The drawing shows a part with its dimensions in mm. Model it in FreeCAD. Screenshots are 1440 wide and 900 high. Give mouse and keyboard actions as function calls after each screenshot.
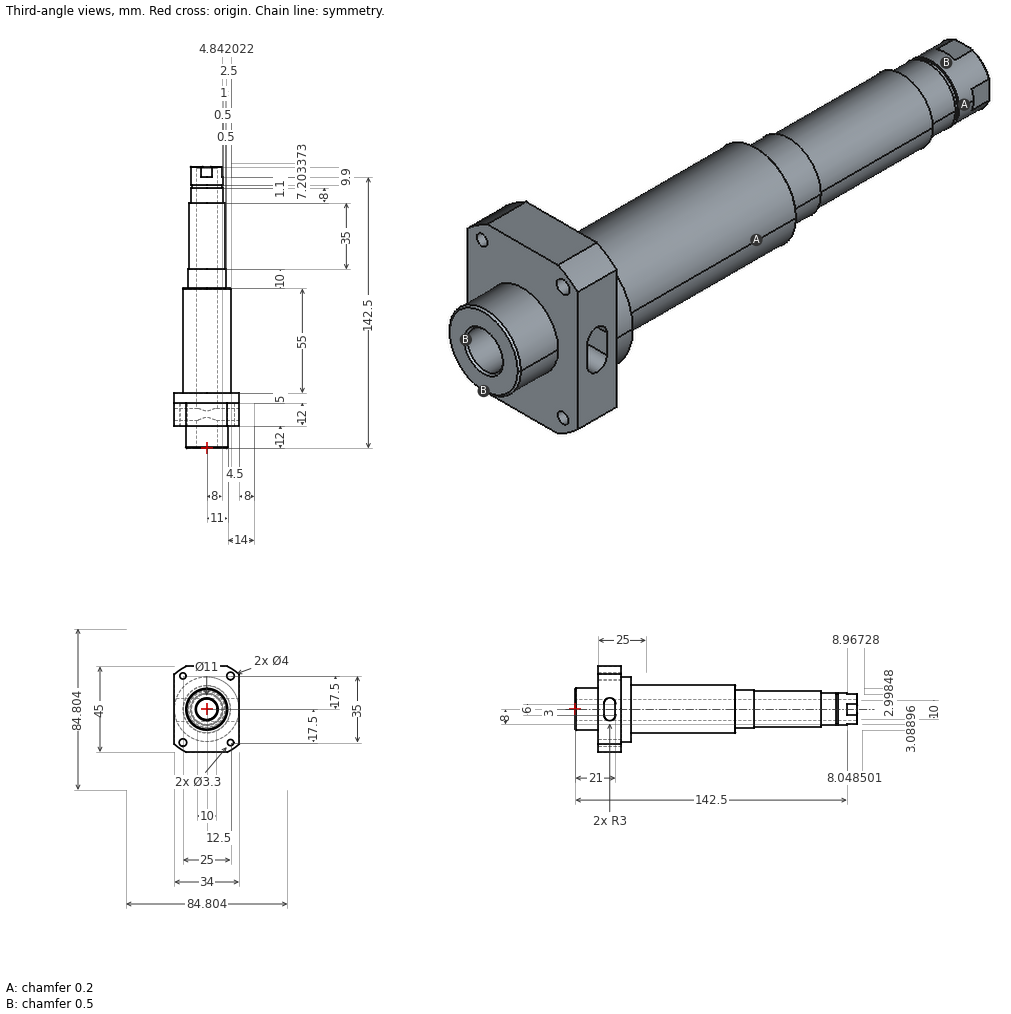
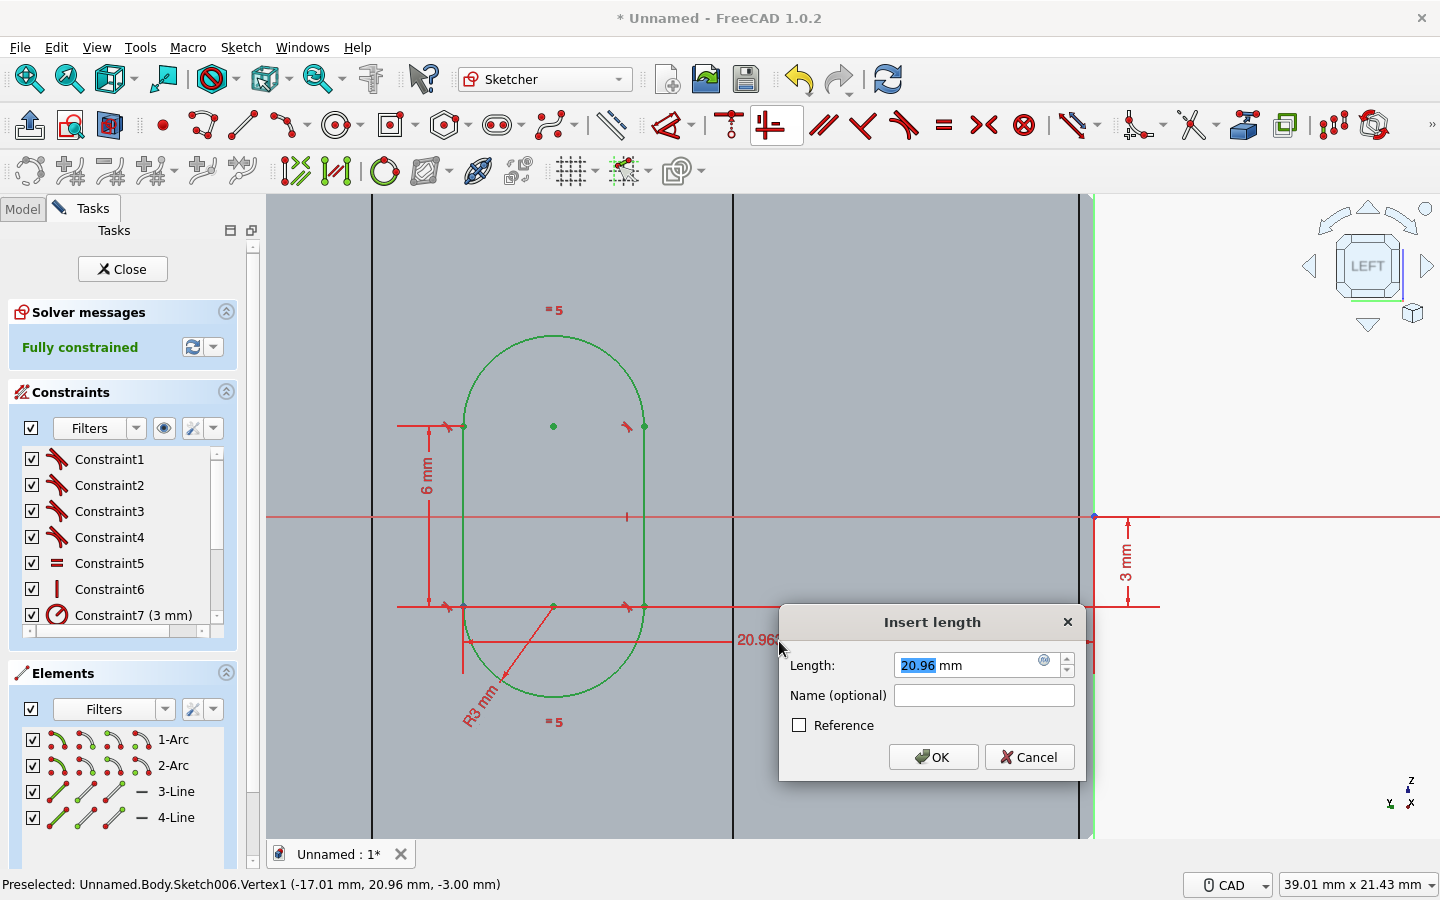
text(21)
key(Return)
key(Escape)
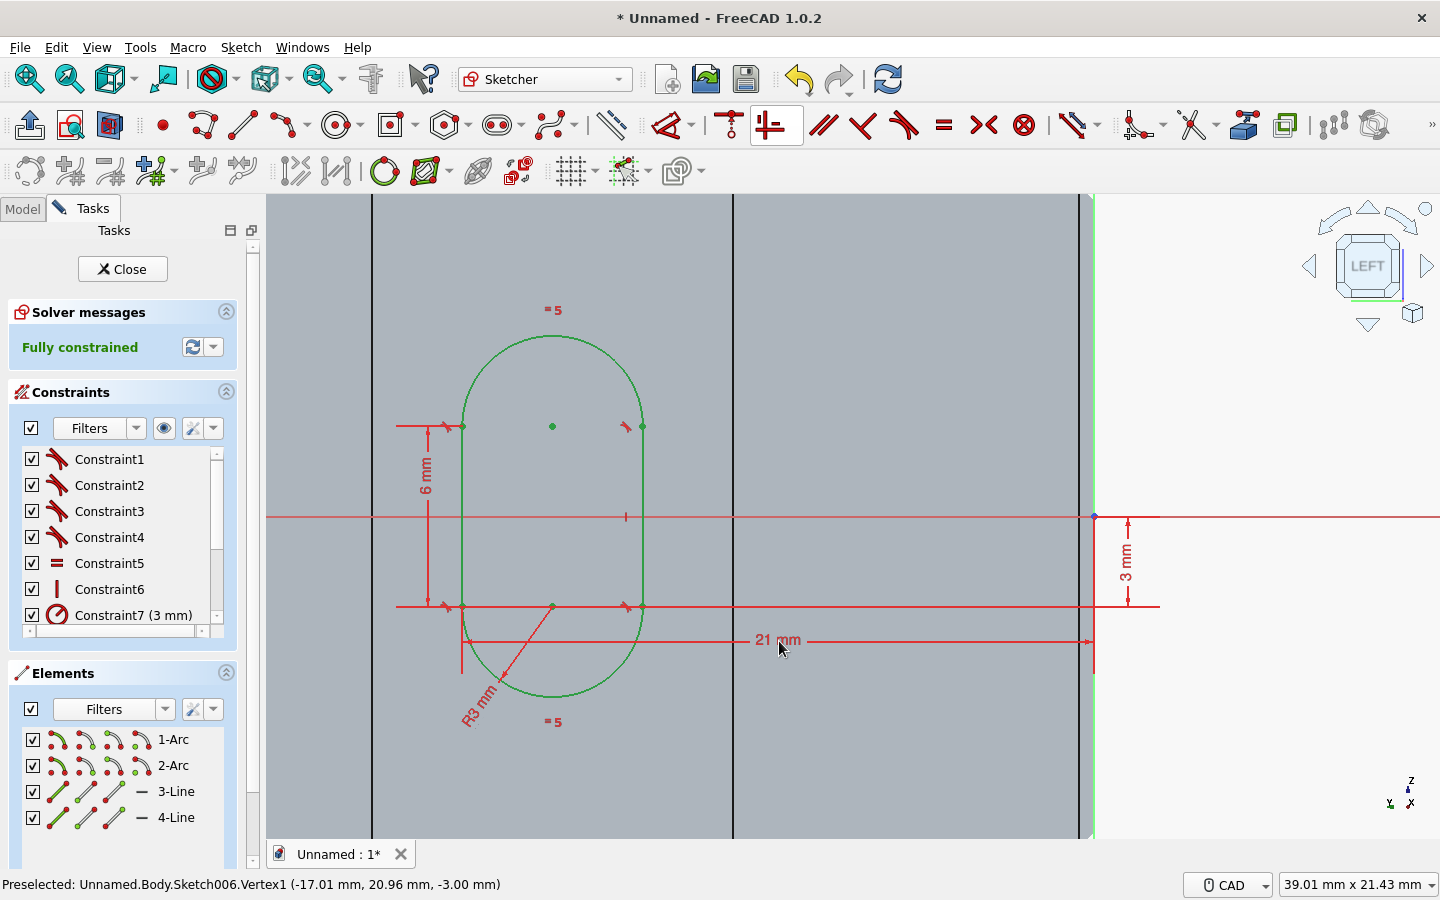
click(123, 269)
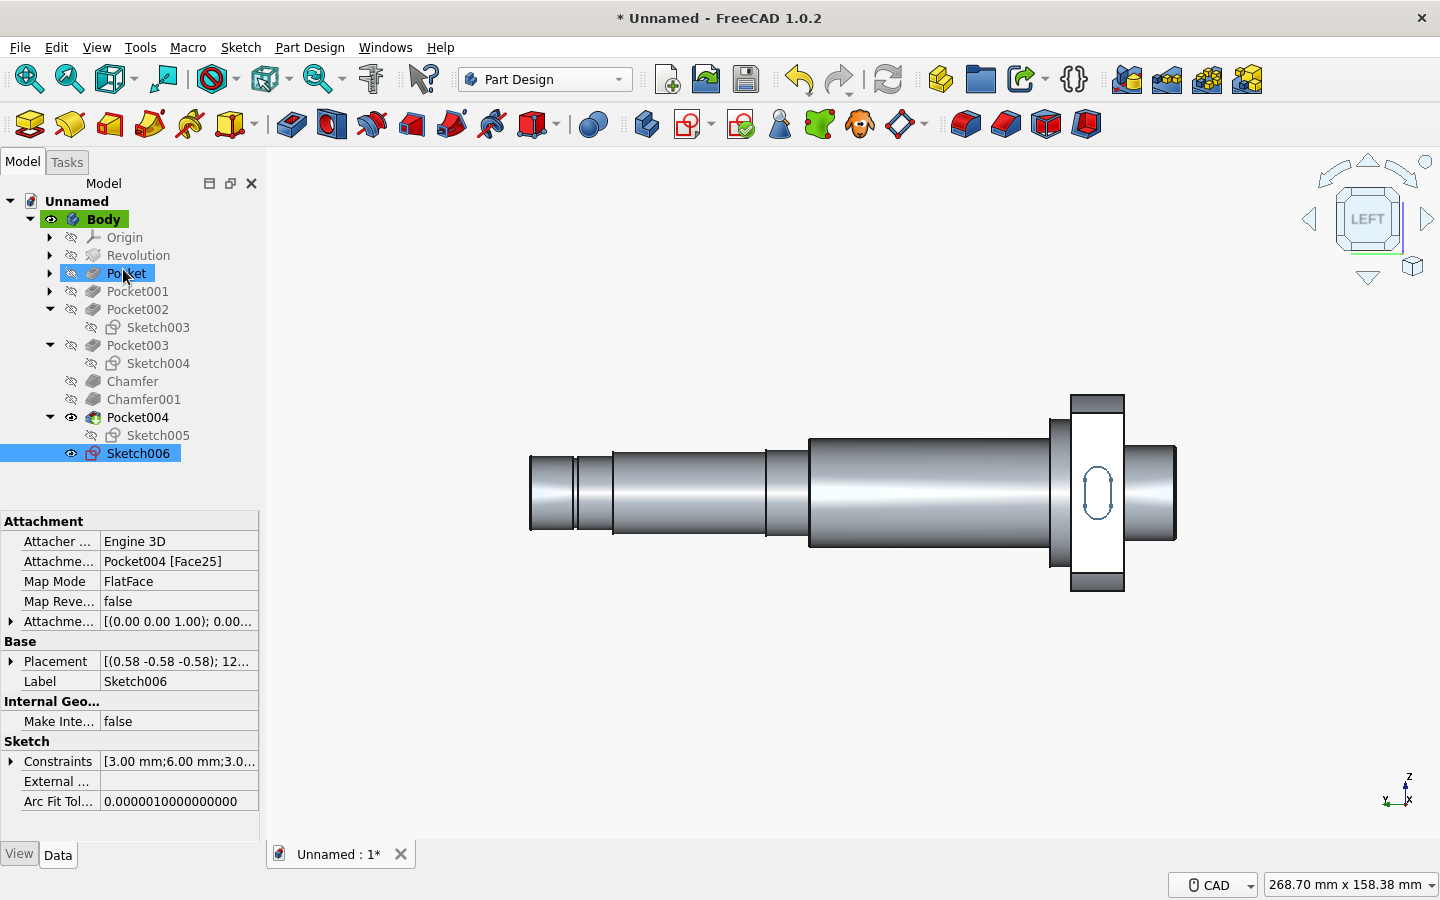
click(292, 124)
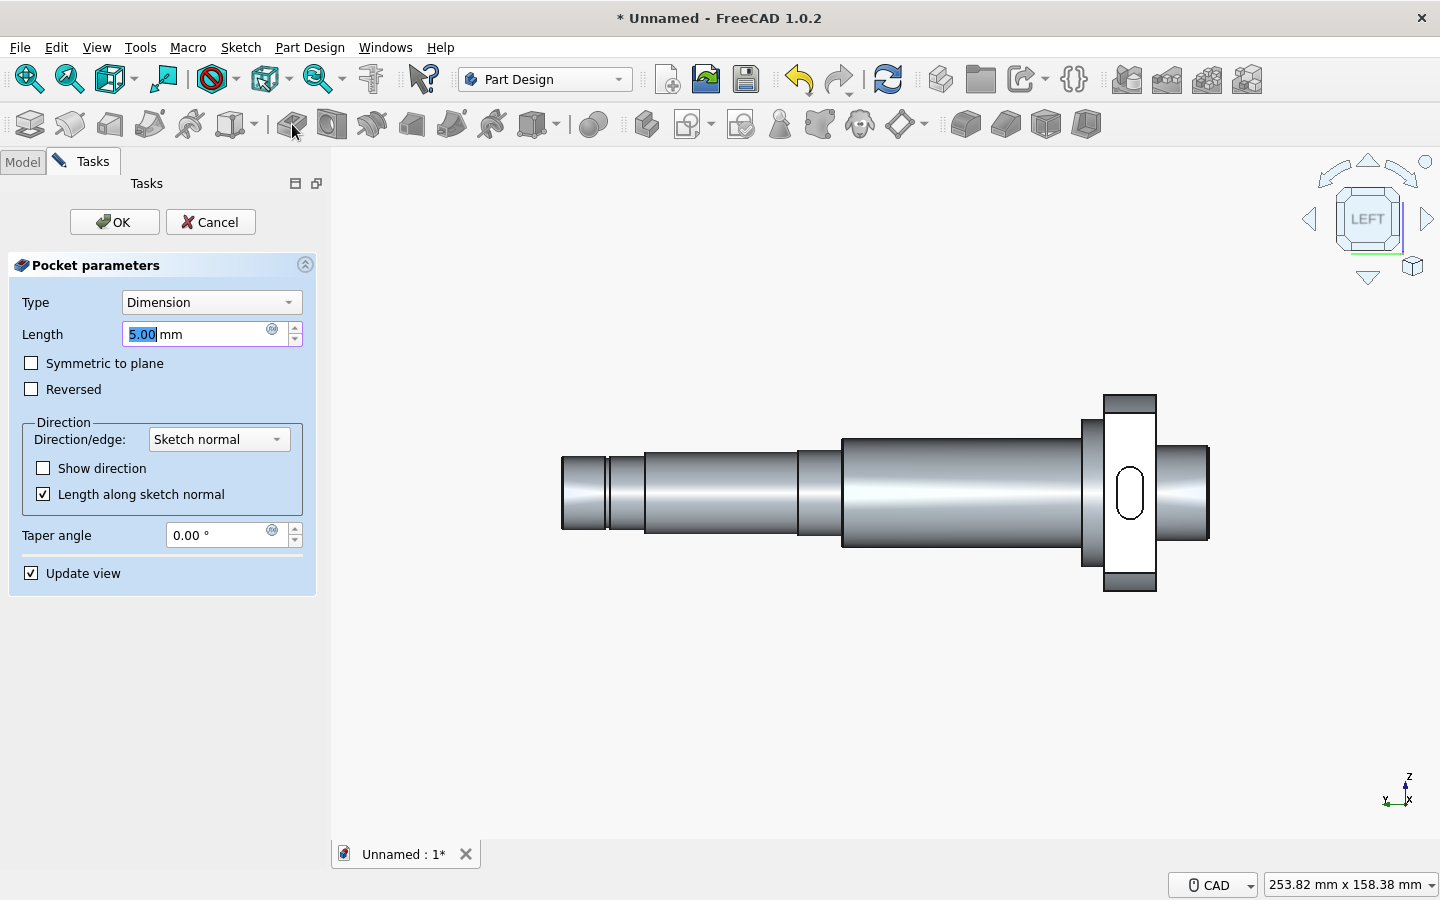
click(212, 302)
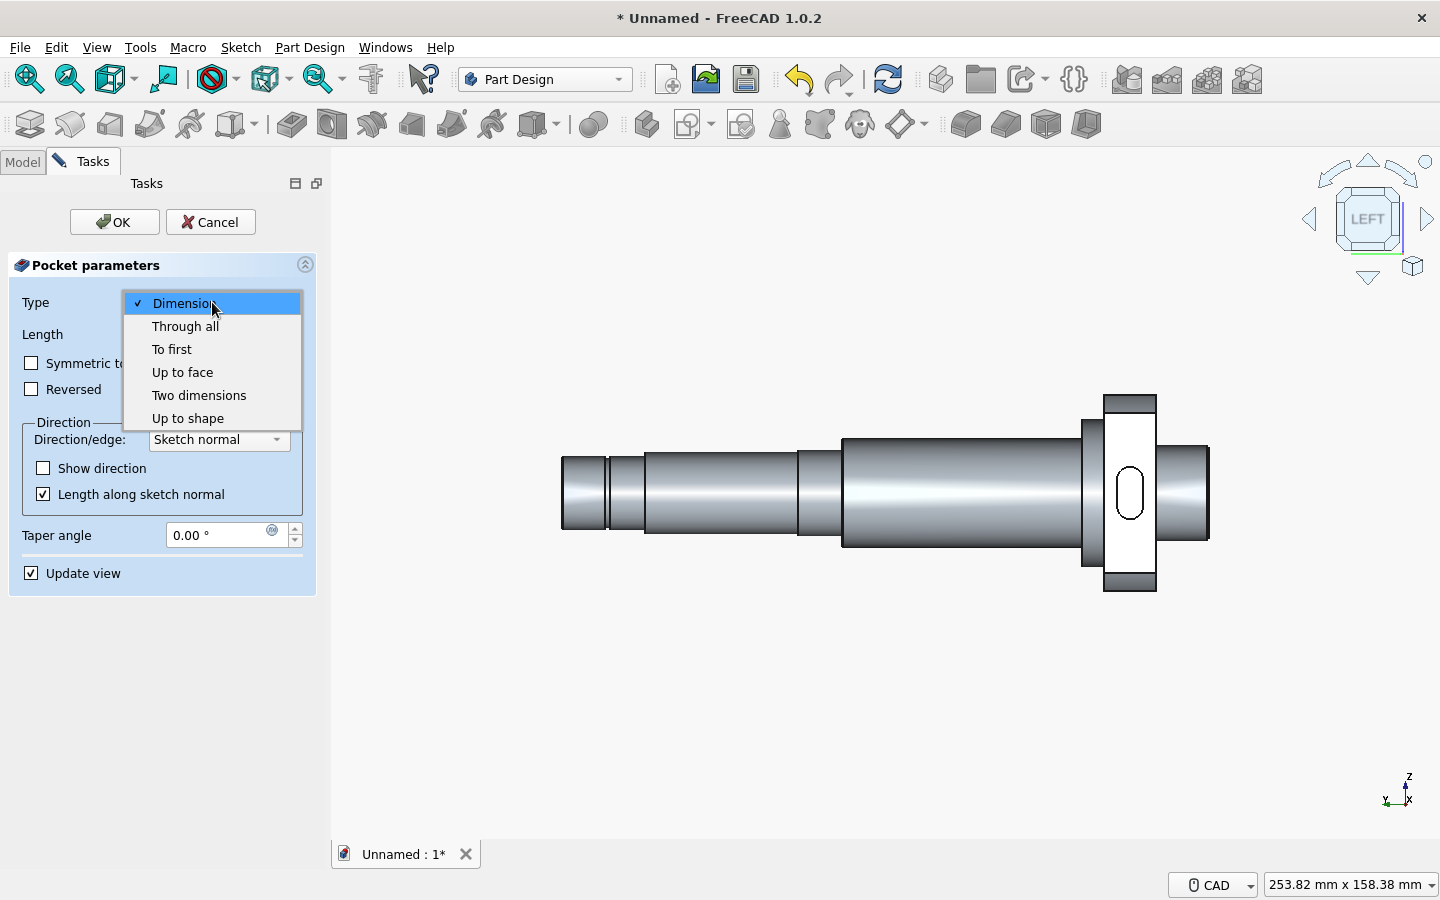
click(212, 326)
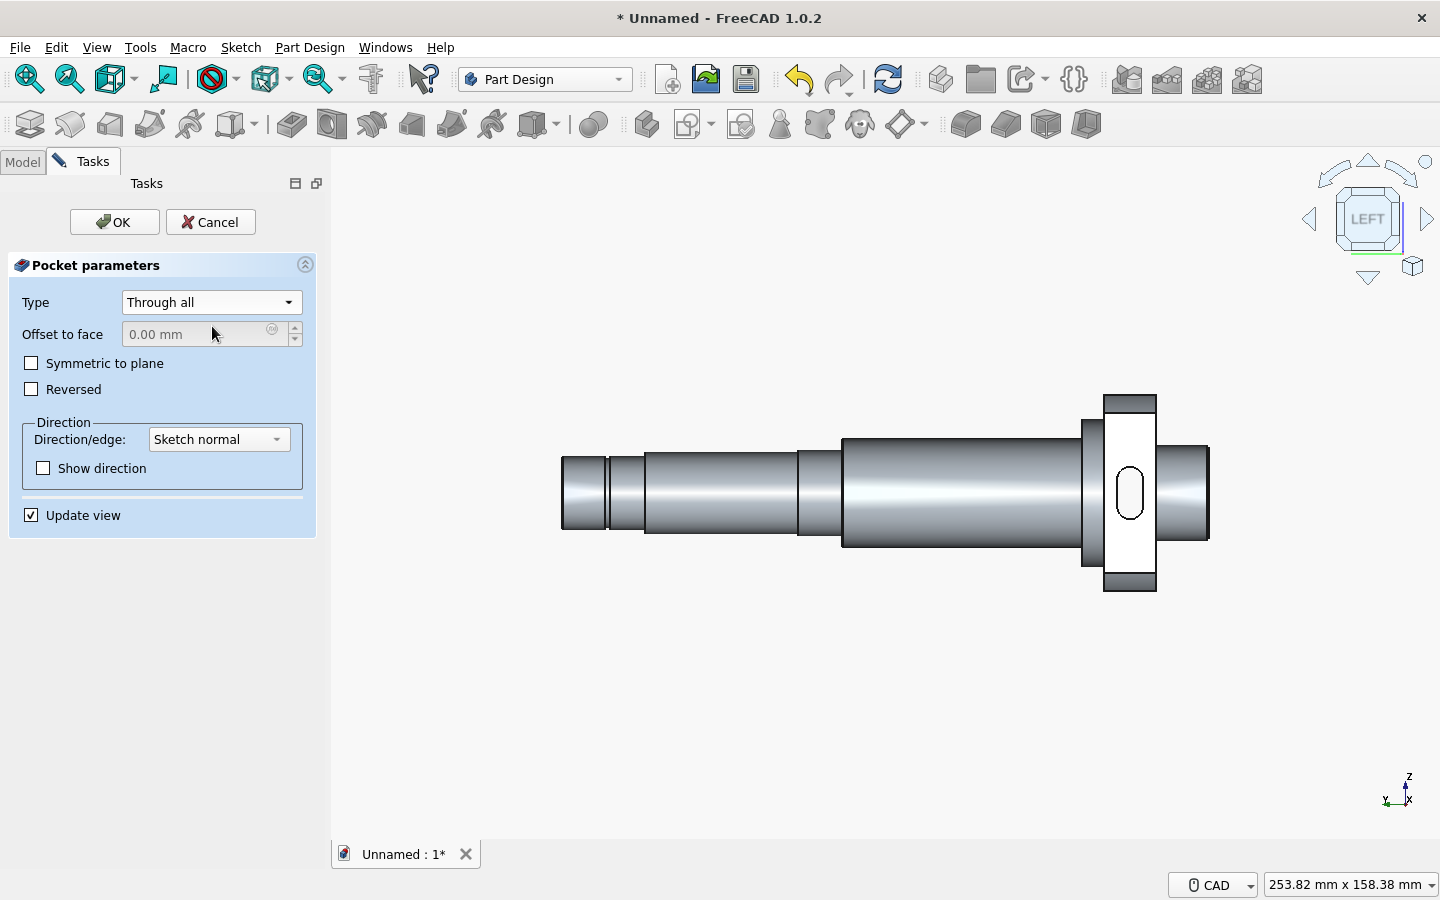
click(115, 222)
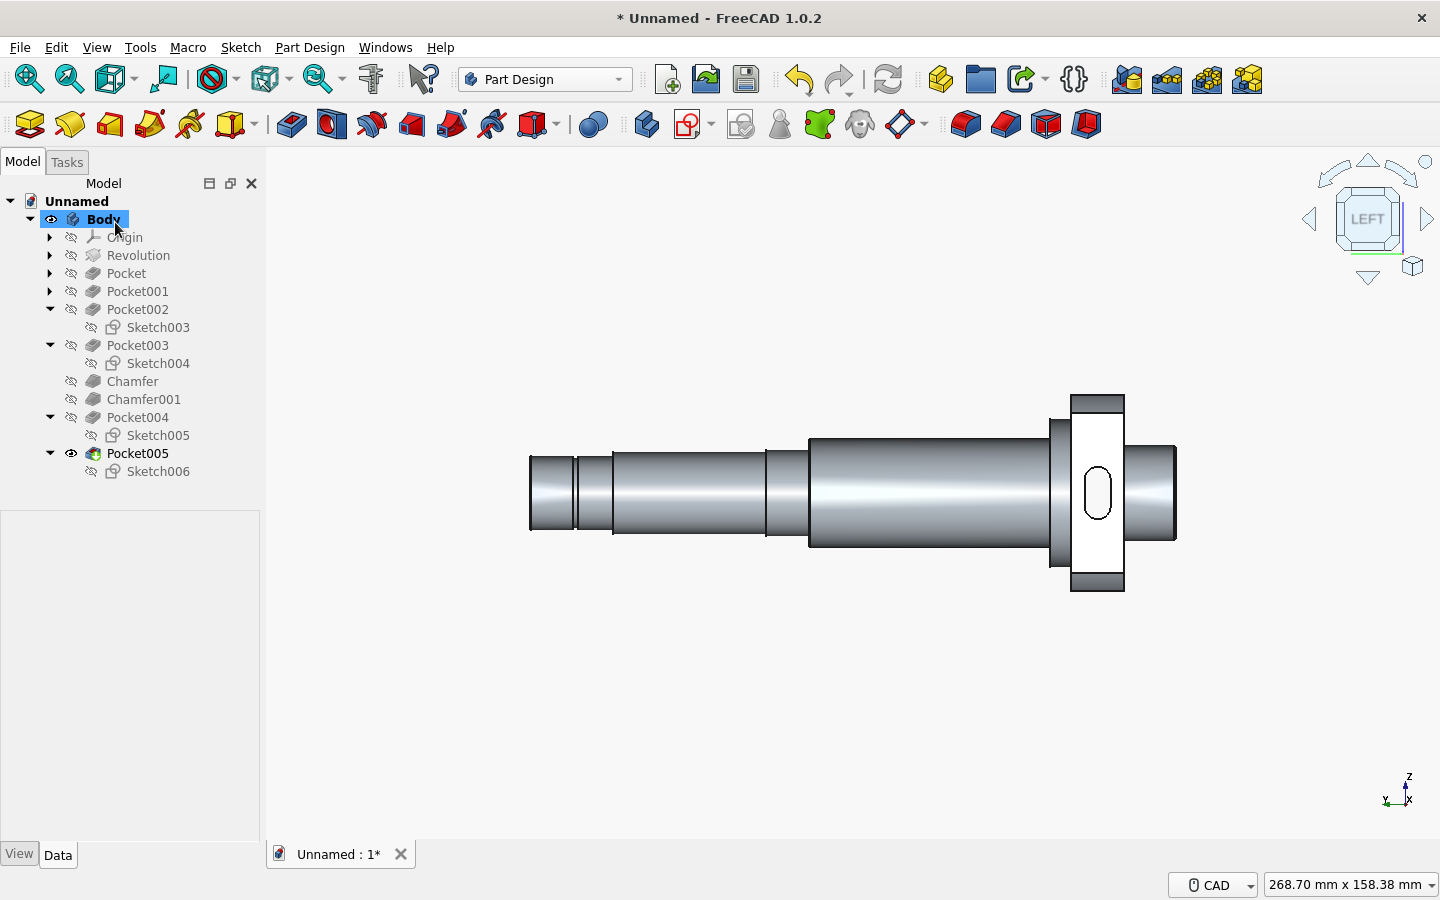
click(688, 124)